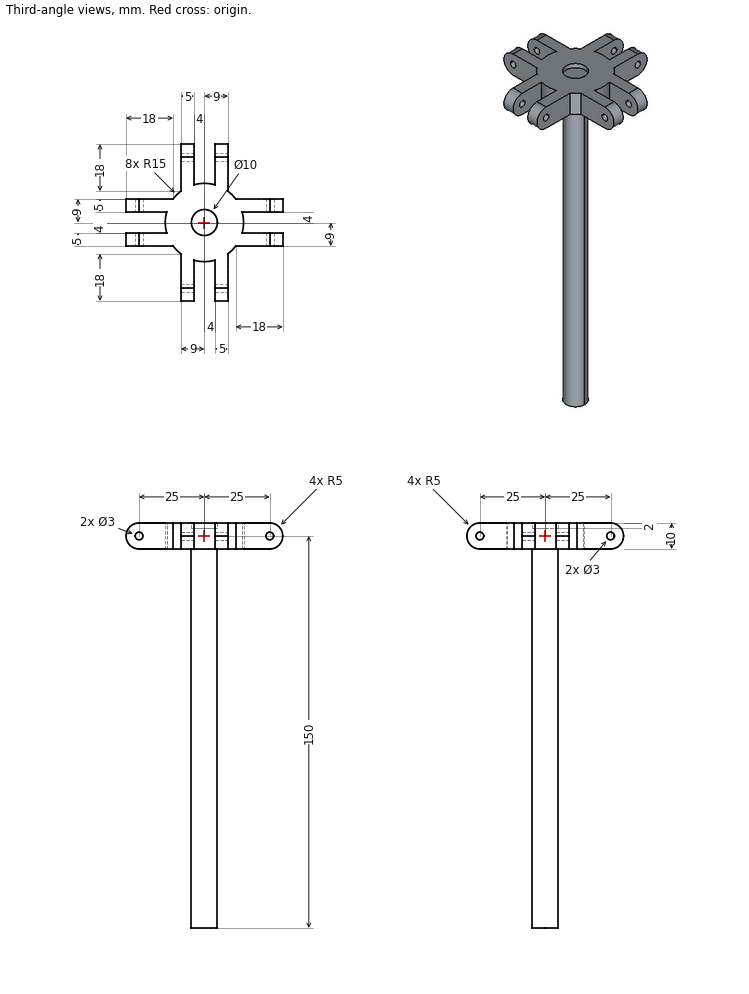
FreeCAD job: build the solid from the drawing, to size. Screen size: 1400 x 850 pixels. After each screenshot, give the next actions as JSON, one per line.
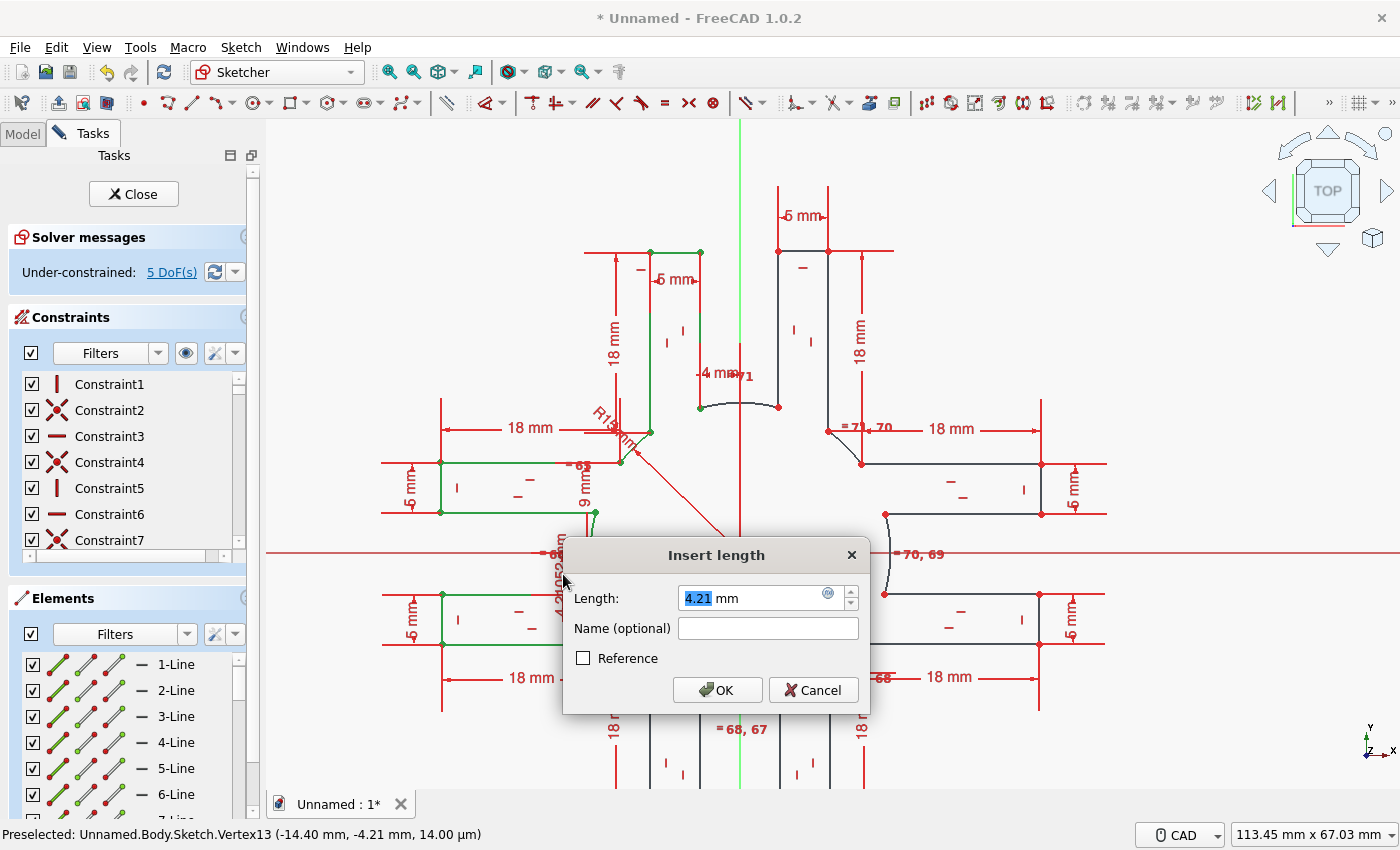
{"action": "type", "text": "4"}
{"action": "key", "text": "Return"}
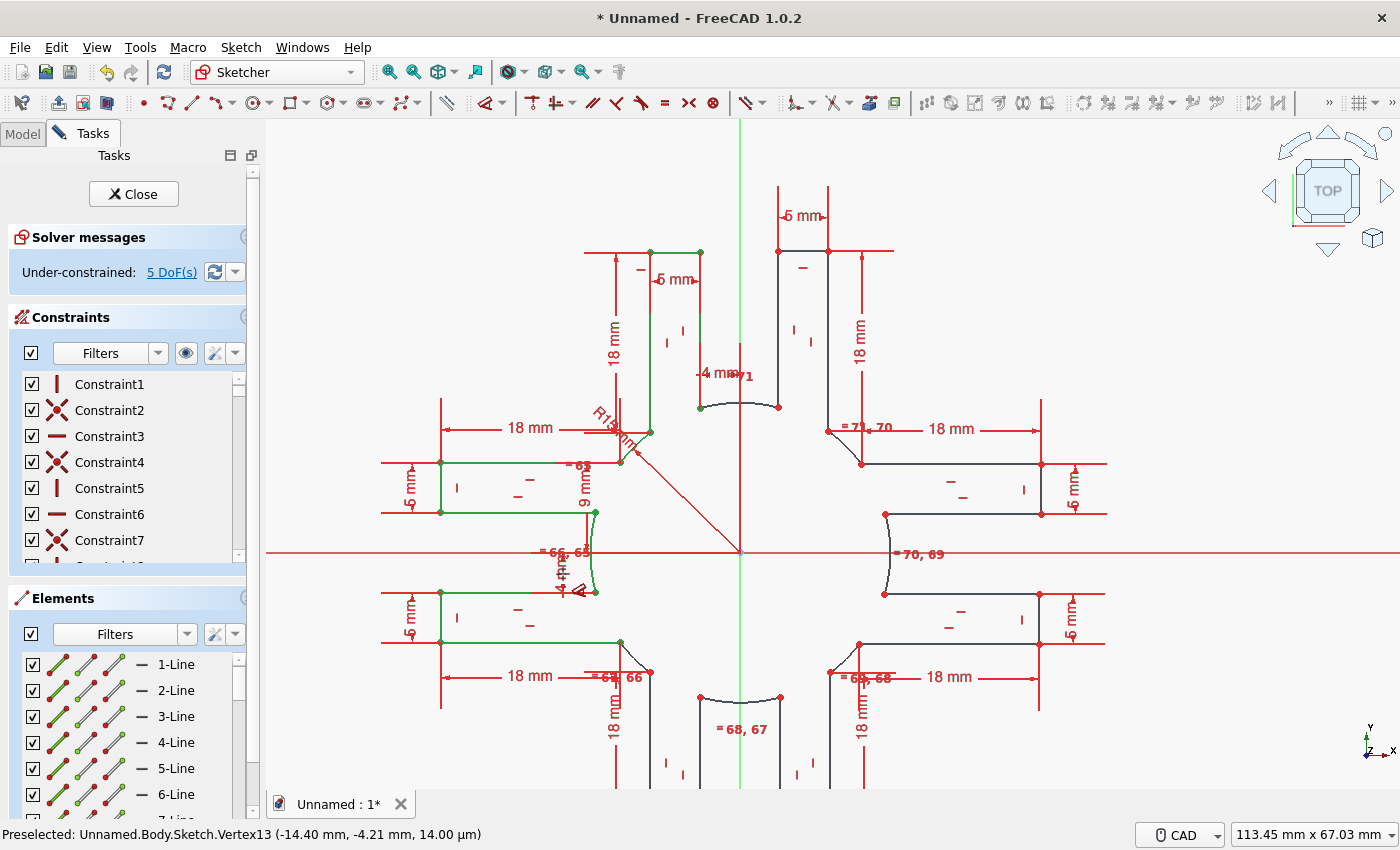
{"action": "left_click", "coordinate": [650, 672]}
{"action": "left_click", "coordinate": [695, 519]}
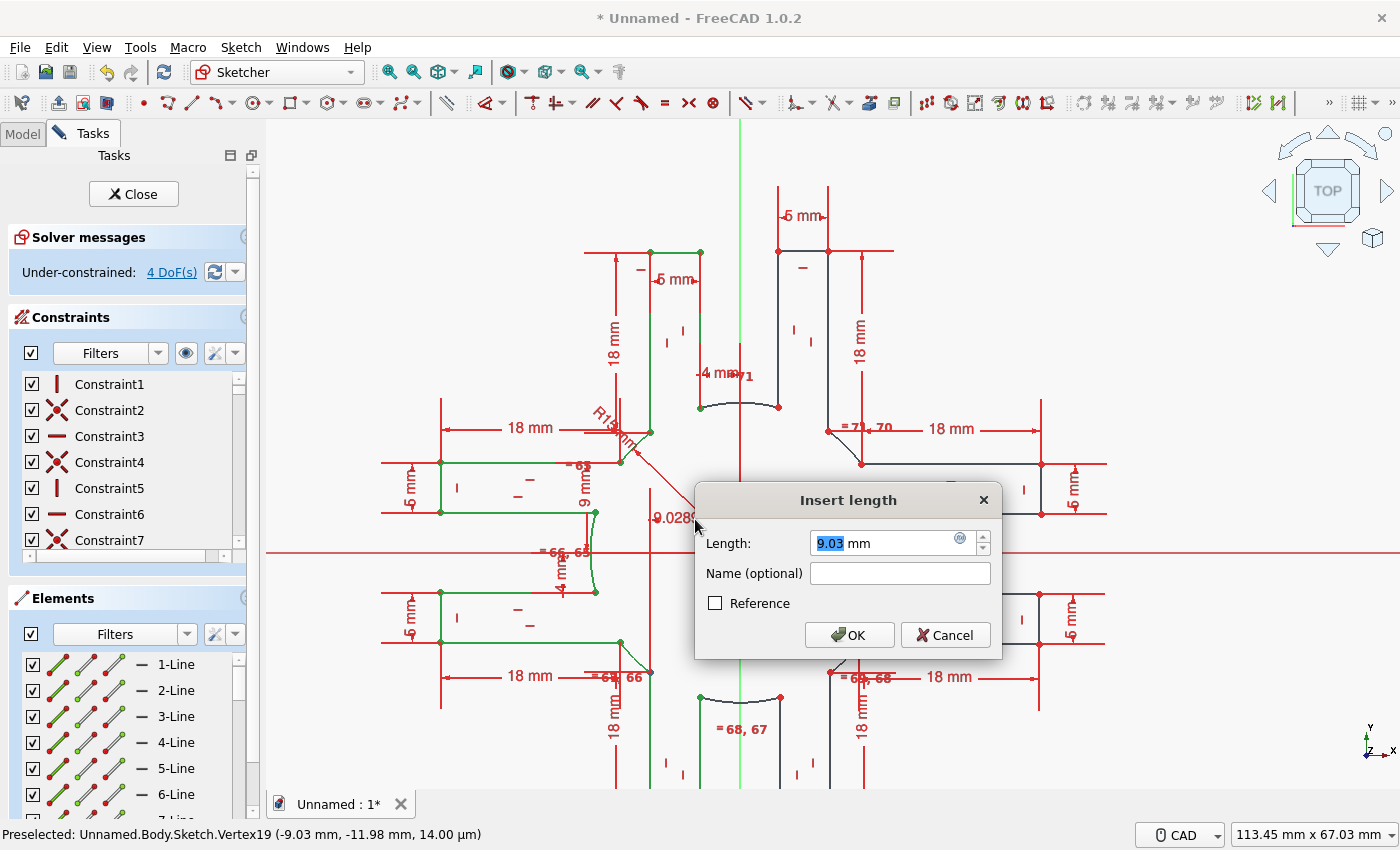
{"action": "type", "text": "9"}
{"action": "key", "text": "Return"}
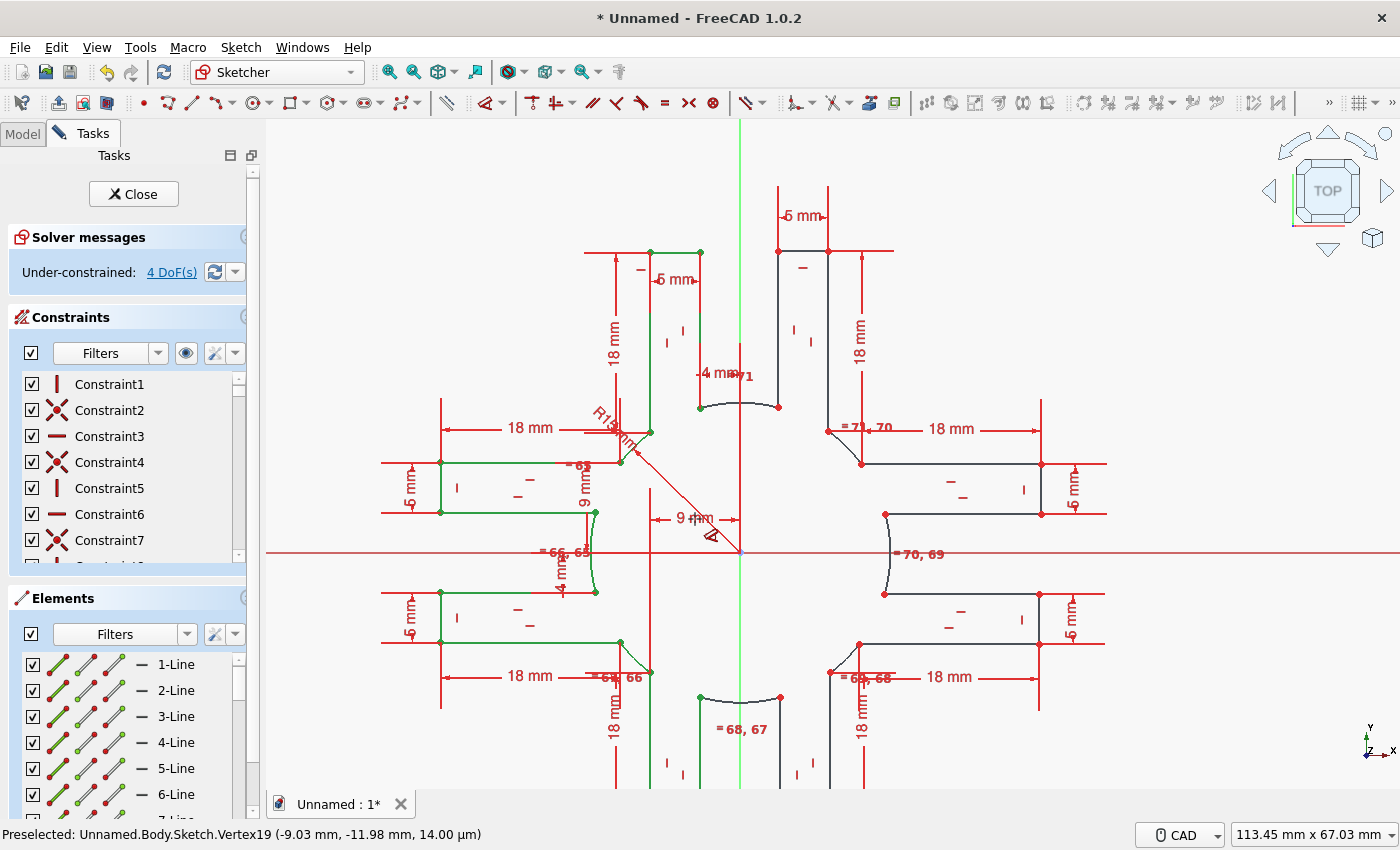
{"action": "left_click", "coordinate": [780, 697]}
{"action": "left_click", "coordinate": [760, 731]}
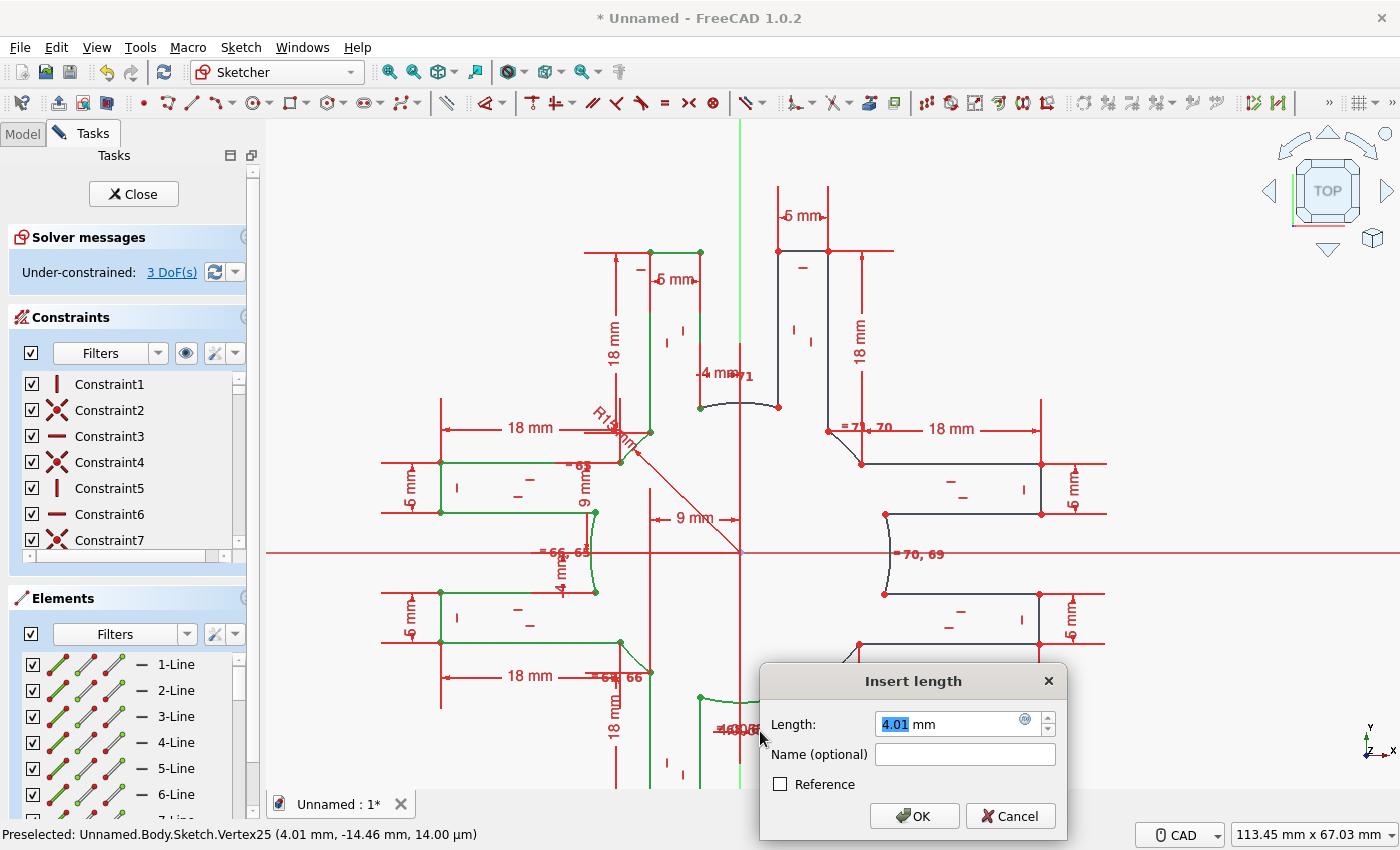
{"action": "type", "text": "4"}
{"action": "key", "text": "Return"}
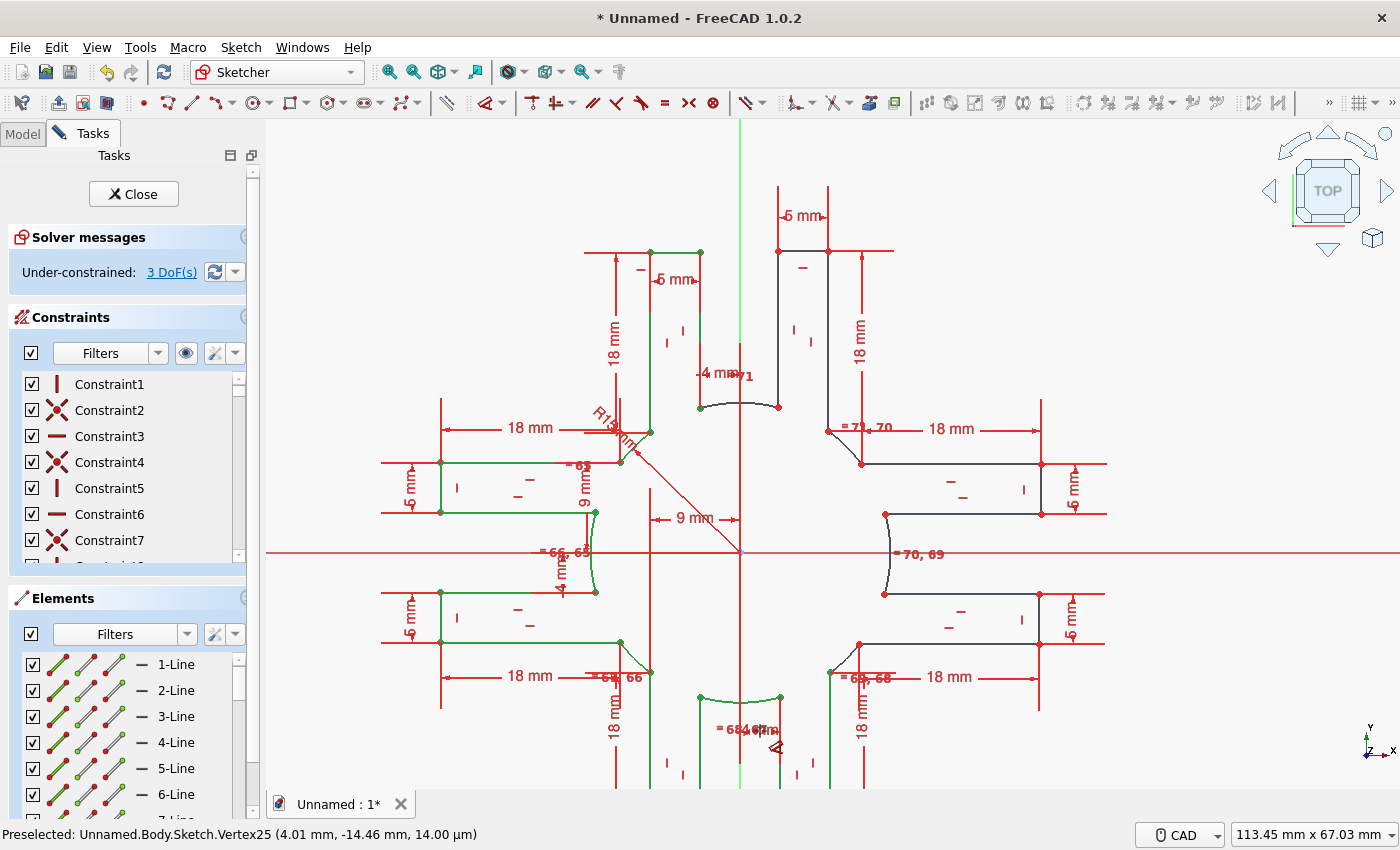
{"action": "left_click", "coordinate": [859, 644]}
{"action": "left_click", "coordinate": [893, 620]}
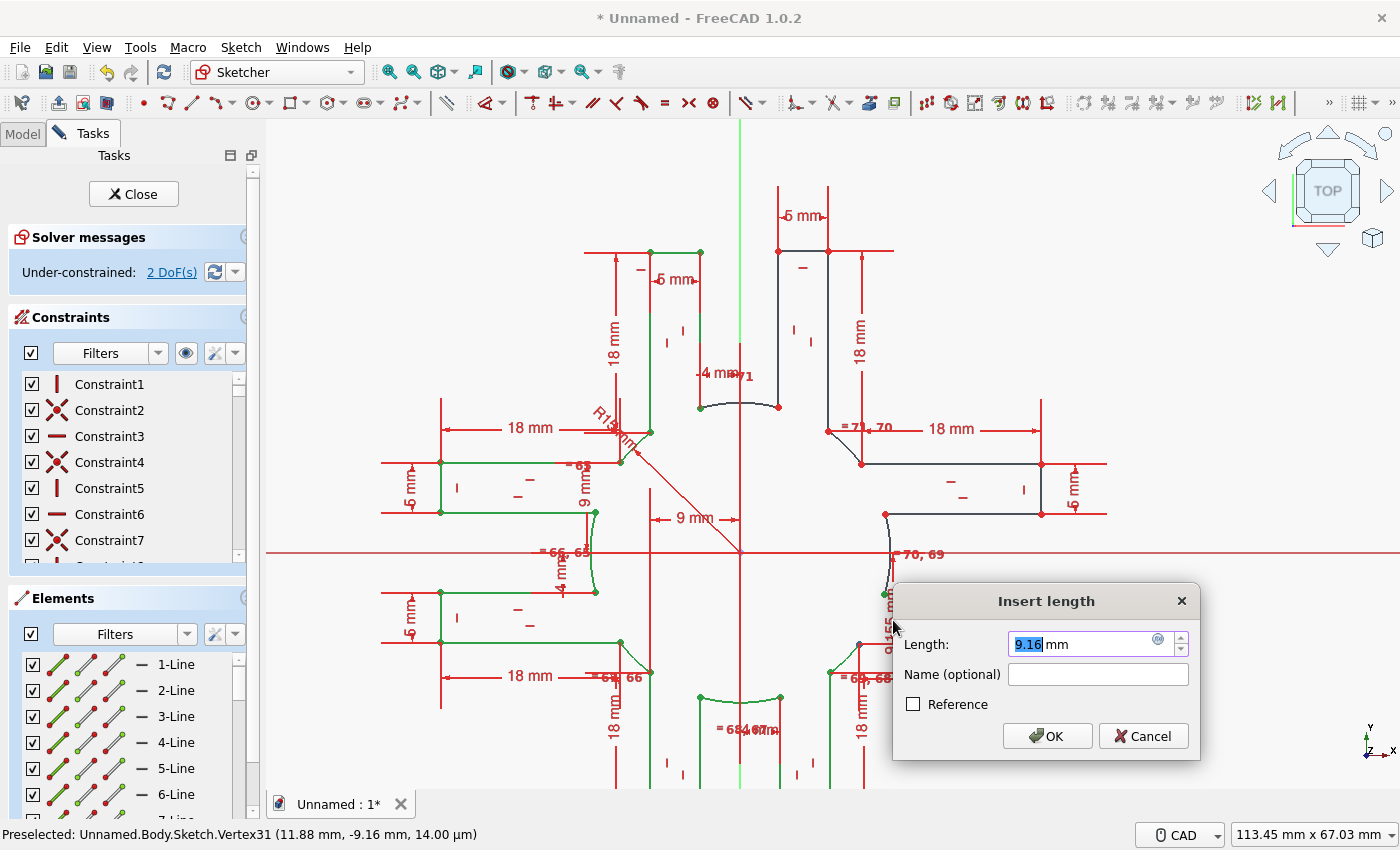
{"action": "type", "text": "9"}
{"action": "key", "text": "Return"}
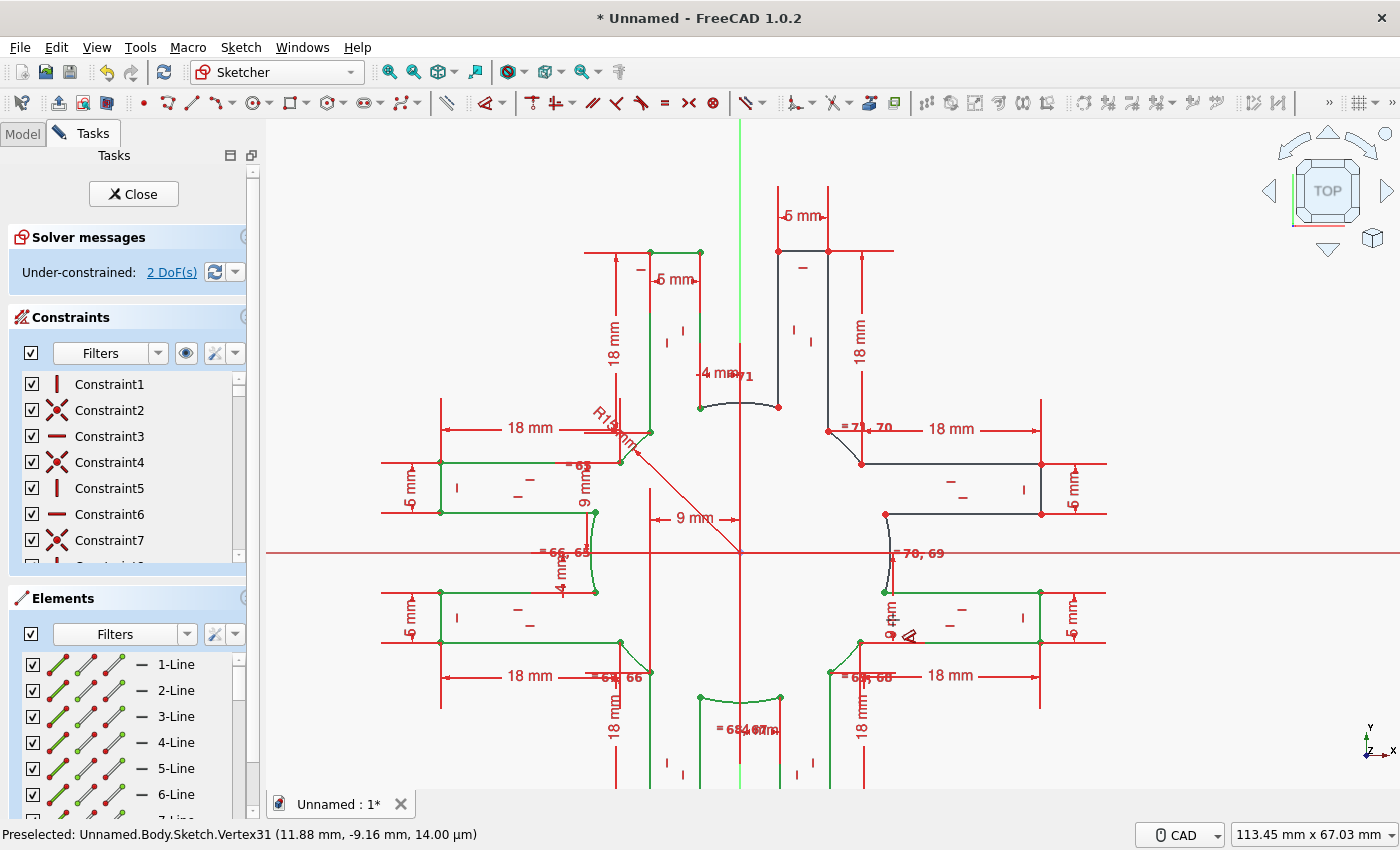
{"action": "left_click", "coordinate": [885, 514]}
{"action": "left_click", "coordinate": [919, 534]}